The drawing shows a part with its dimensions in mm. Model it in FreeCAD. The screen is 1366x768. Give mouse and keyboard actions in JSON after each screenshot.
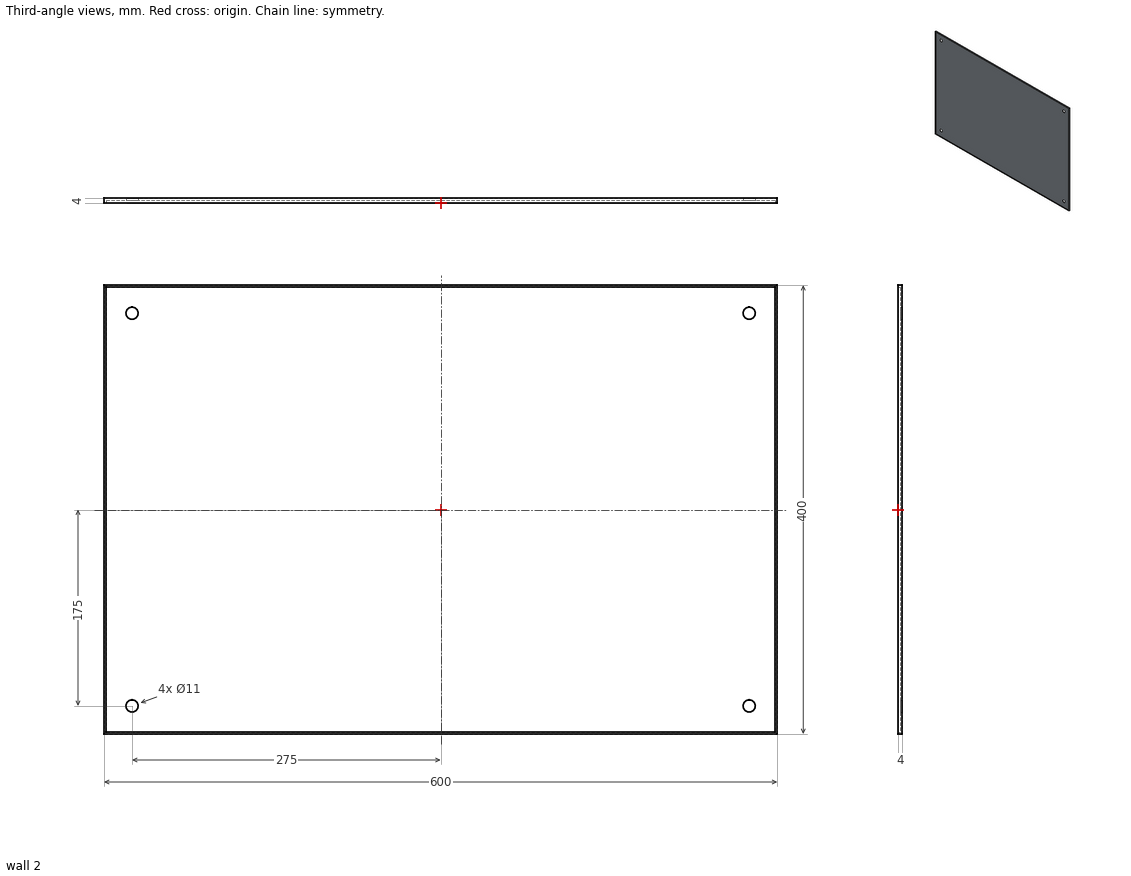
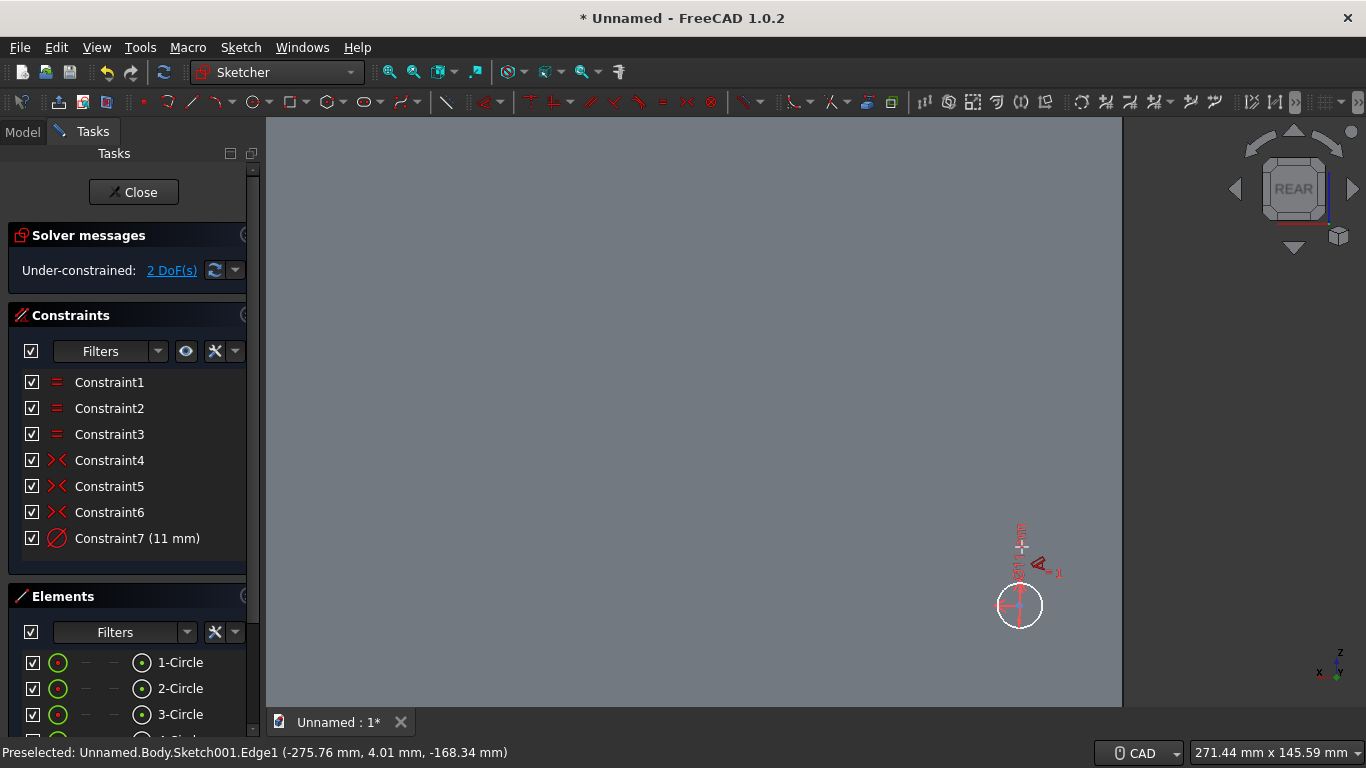
{"action": "scroll", "coordinate": [1022, 580], "scroll_direction": "down", "scroll_amount": 7}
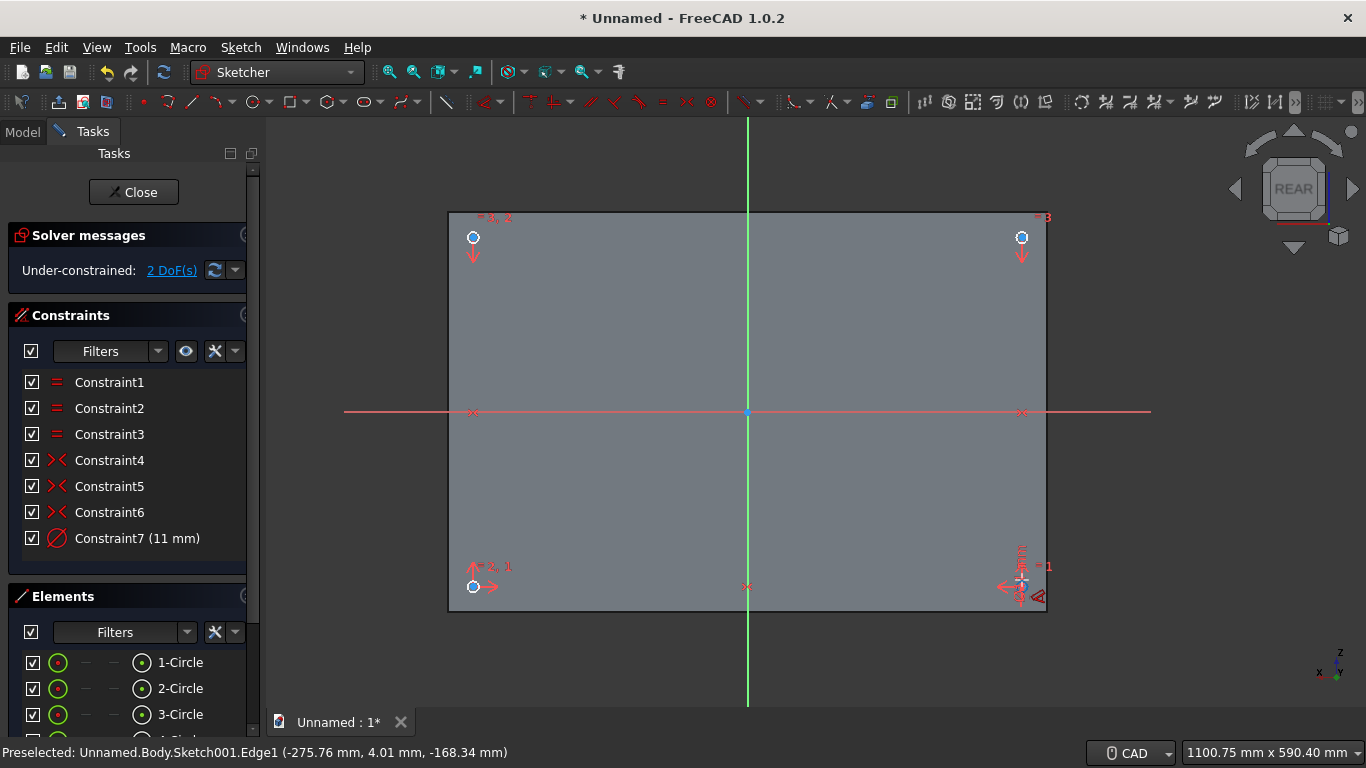
{"action": "left_click", "coordinate": [1022, 587]}
{"action": "left_click", "coordinate": [885, 621]}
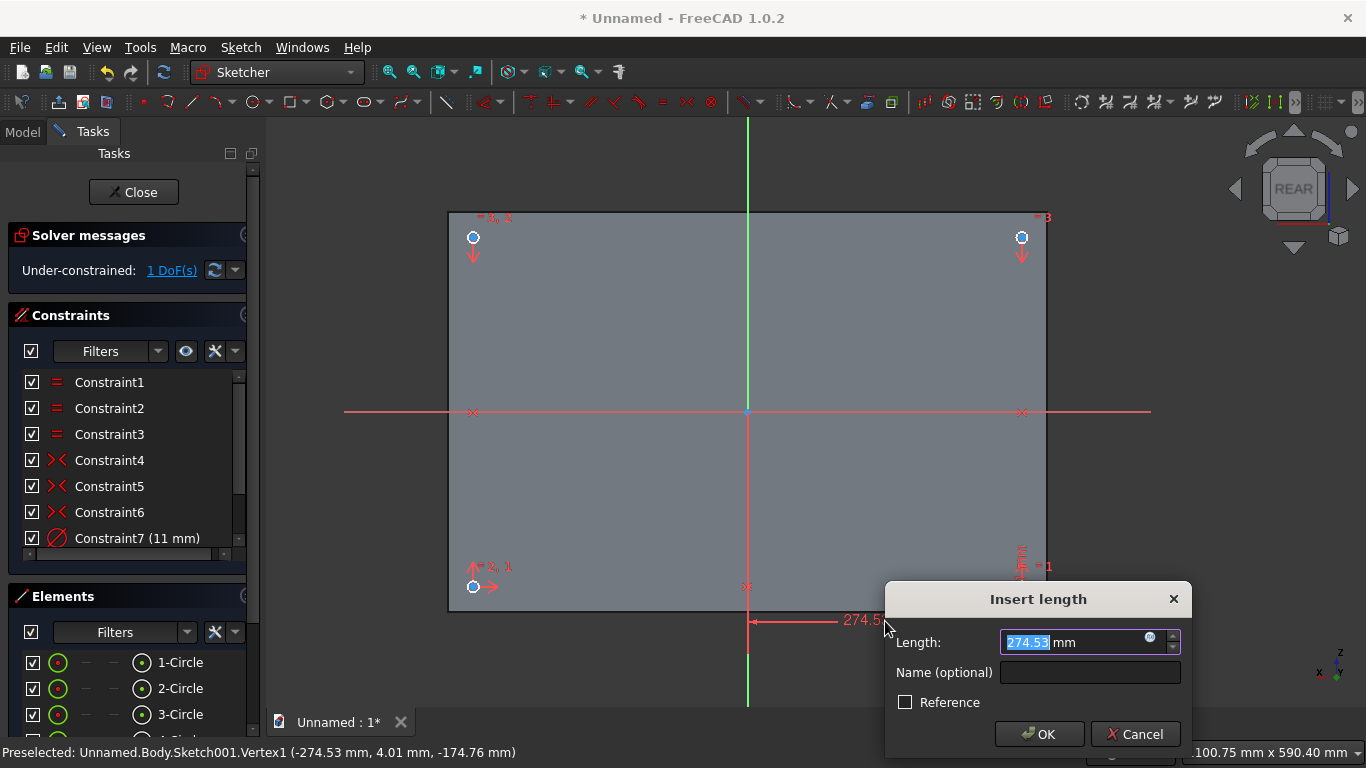
{"action": "type", "text": "275"}
{"action": "key", "text": "Return"}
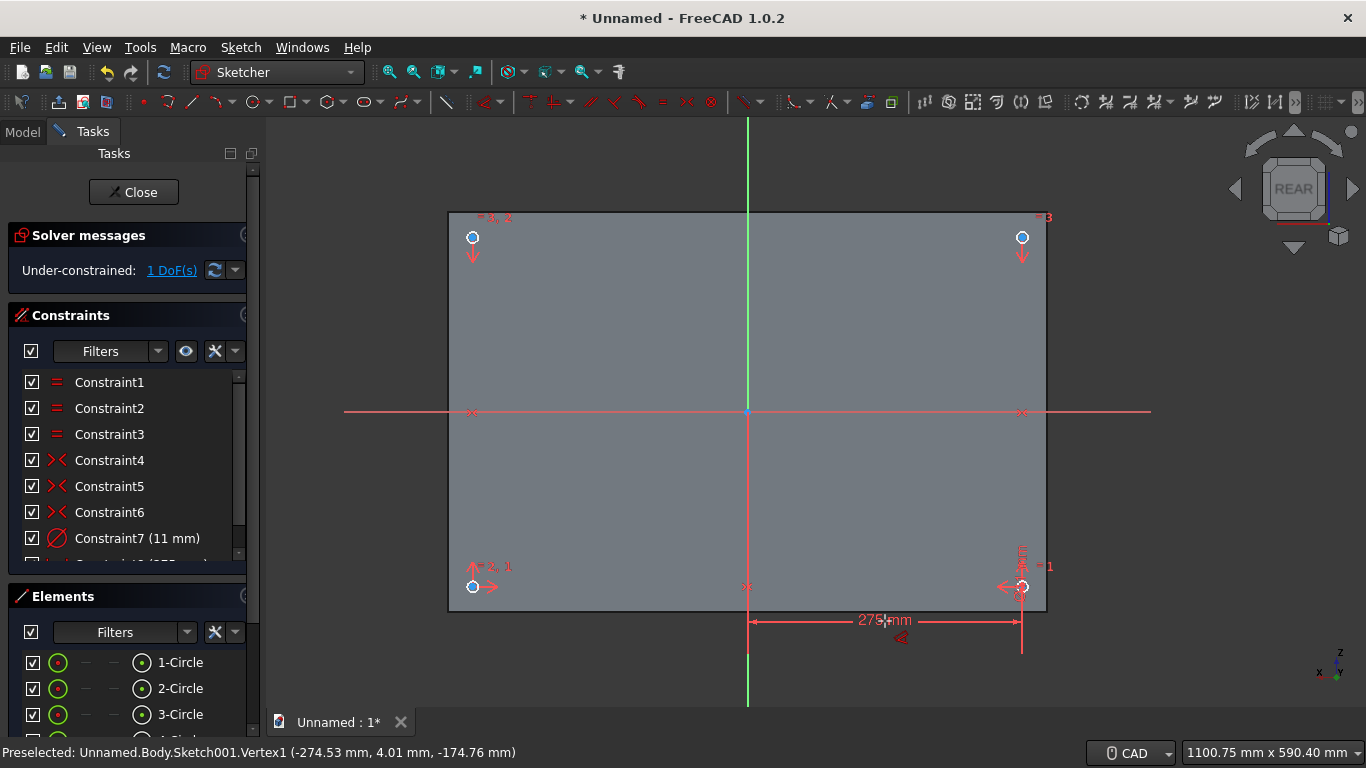
{"action": "left_click", "coordinate": [1022, 587]}
{"action": "left_click", "coordinate": [1056, 500]}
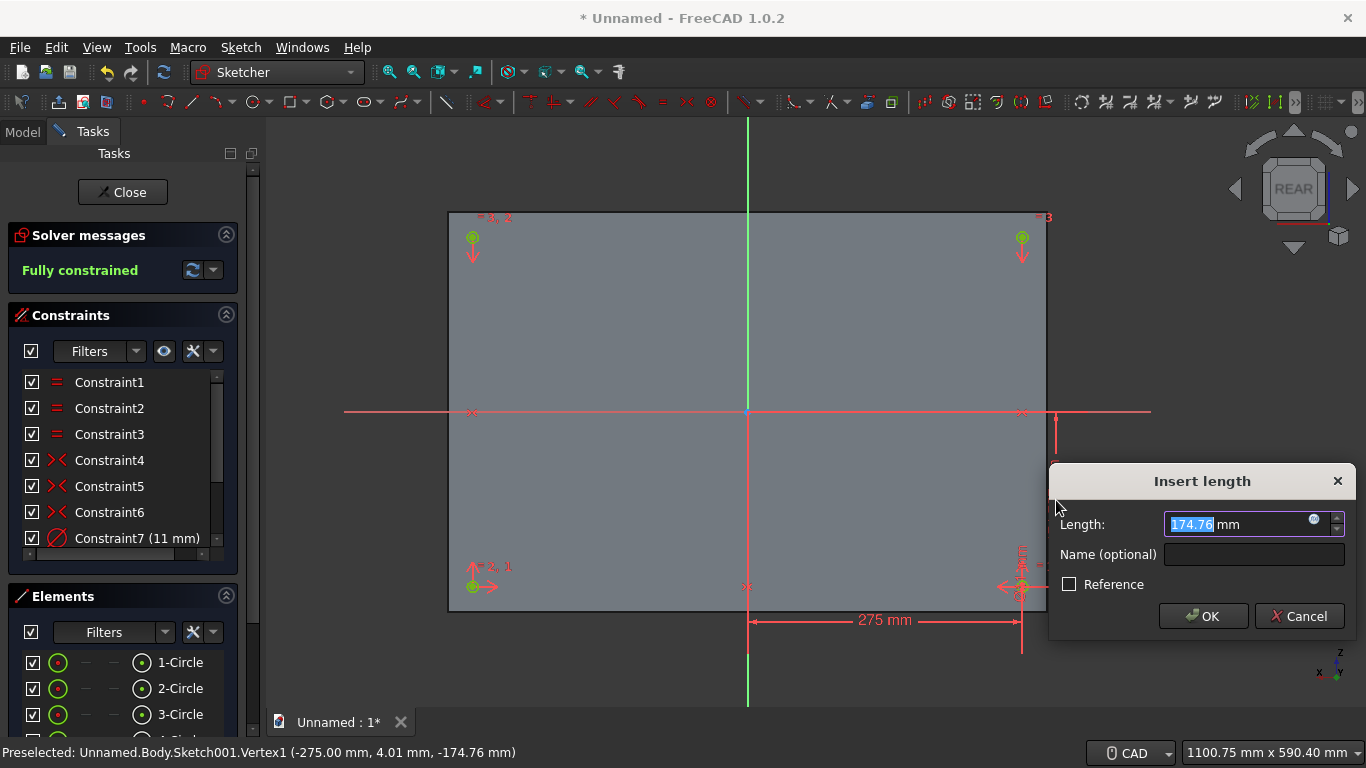
{"action": "type", "text": "175"}
{"action": "key", "text": "Return"}
{"action": "key", "text": "Escape"}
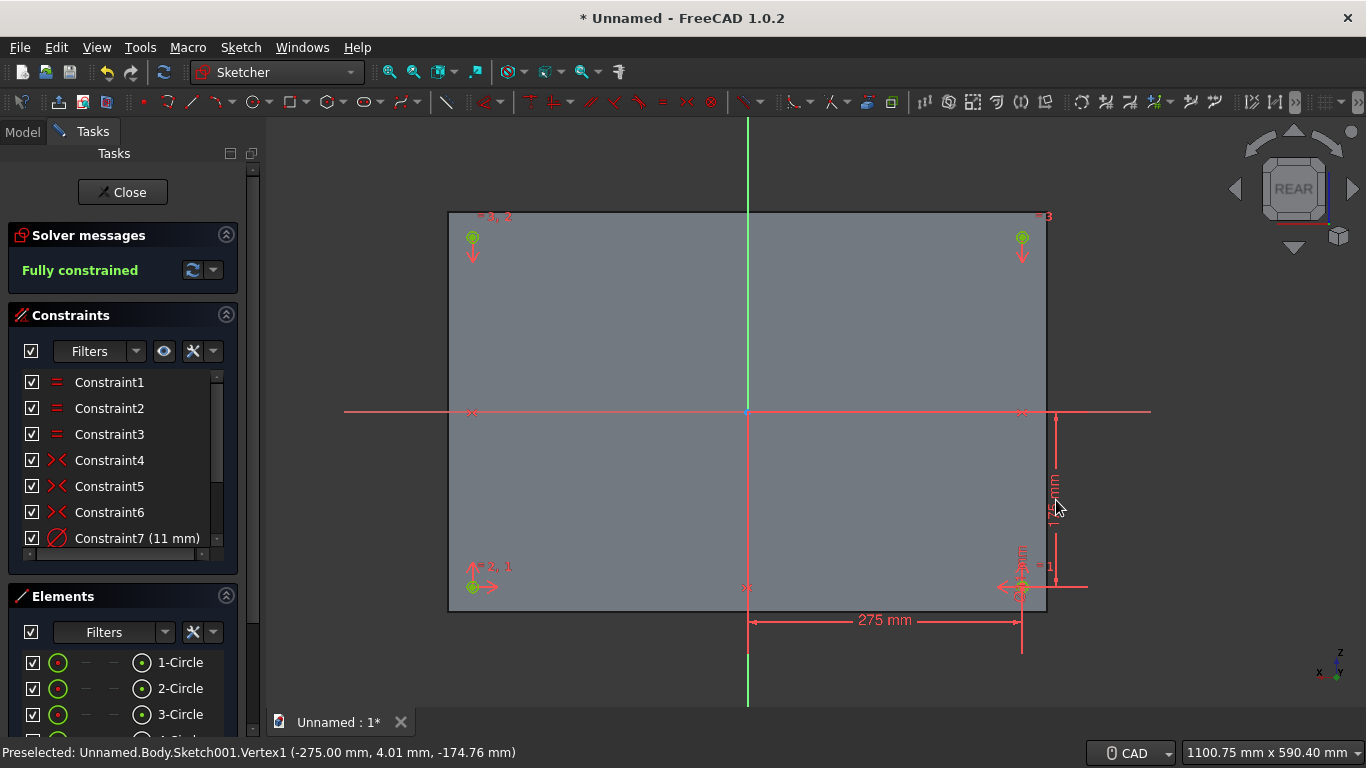
{"action": "left_click", "coordinate": [123, 192]}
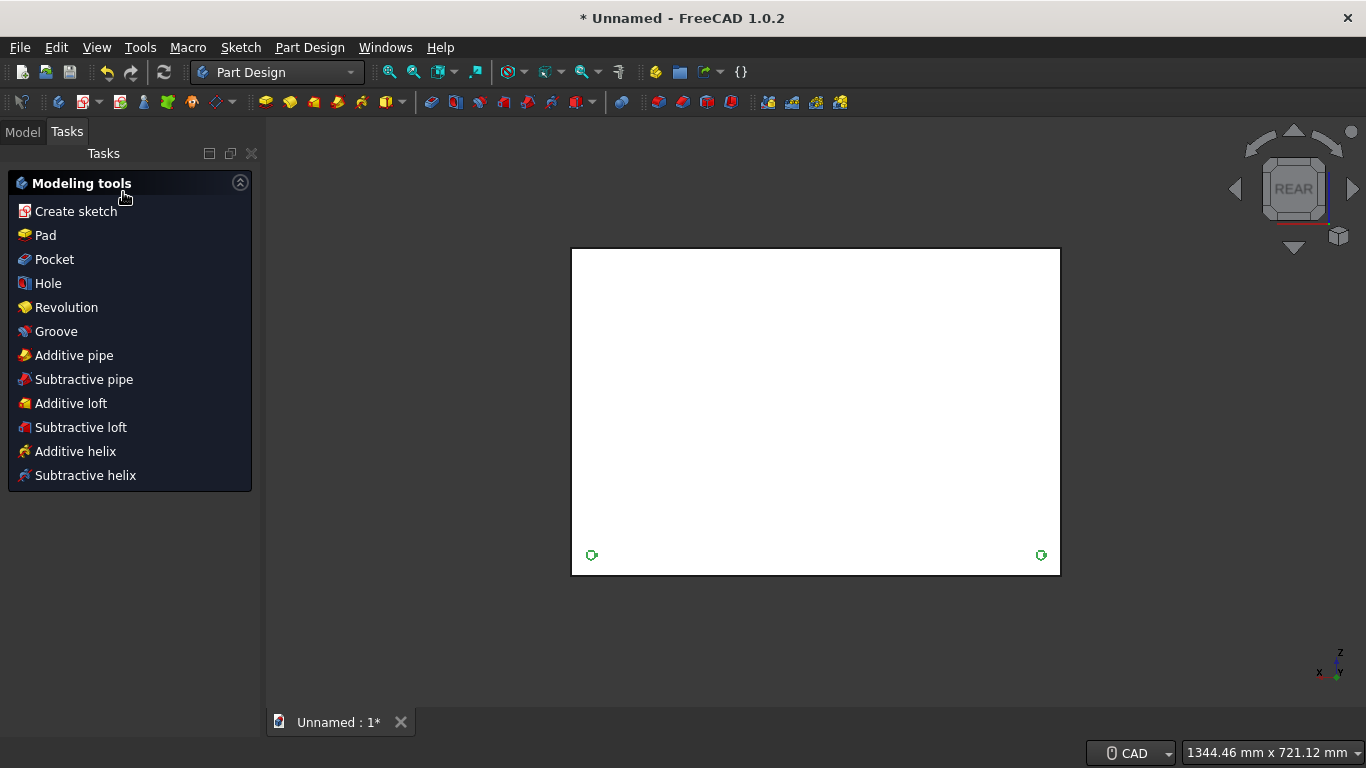
{"action": "left_click", "coordinate": [432, 102]}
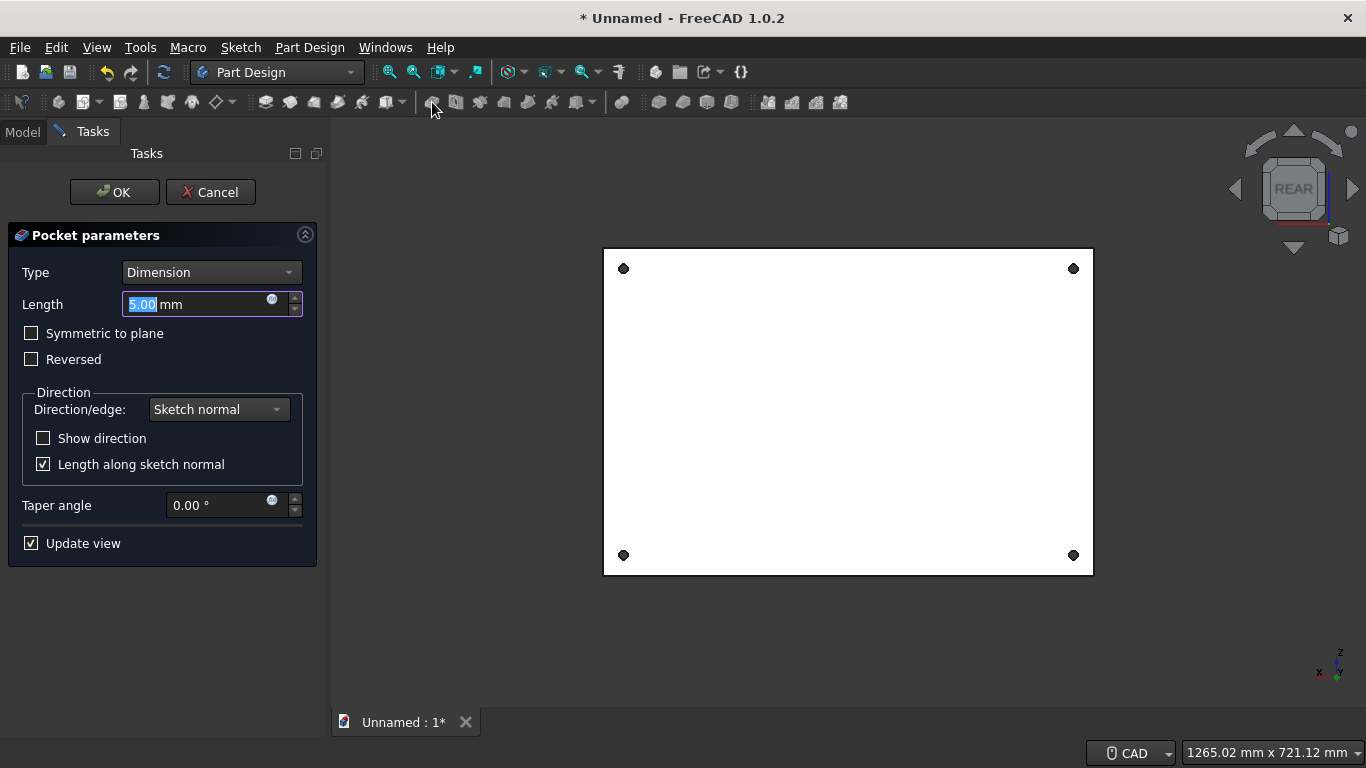
{"action": "type", "text": "4"}
{"action": "key", "text": "Tab"}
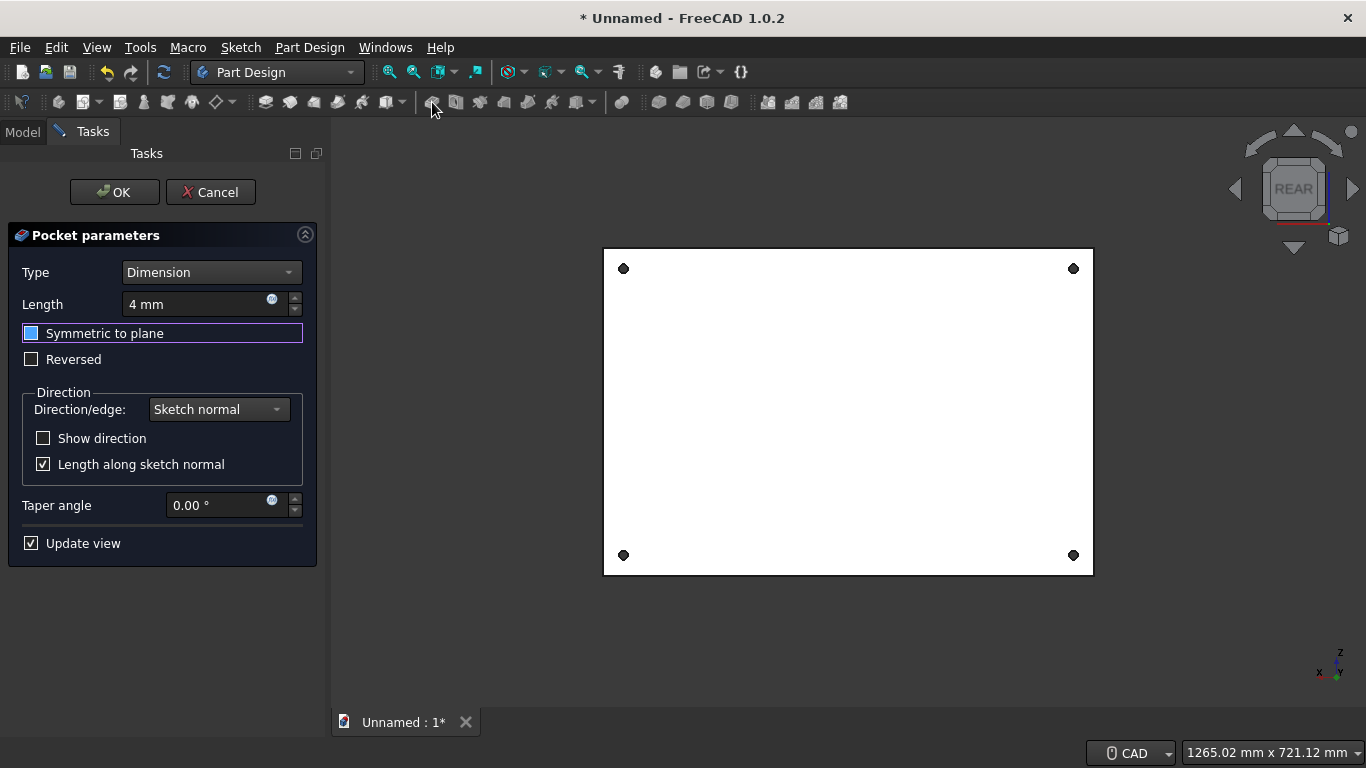
{"action": "left_click", "coordinate": [115, 192]}